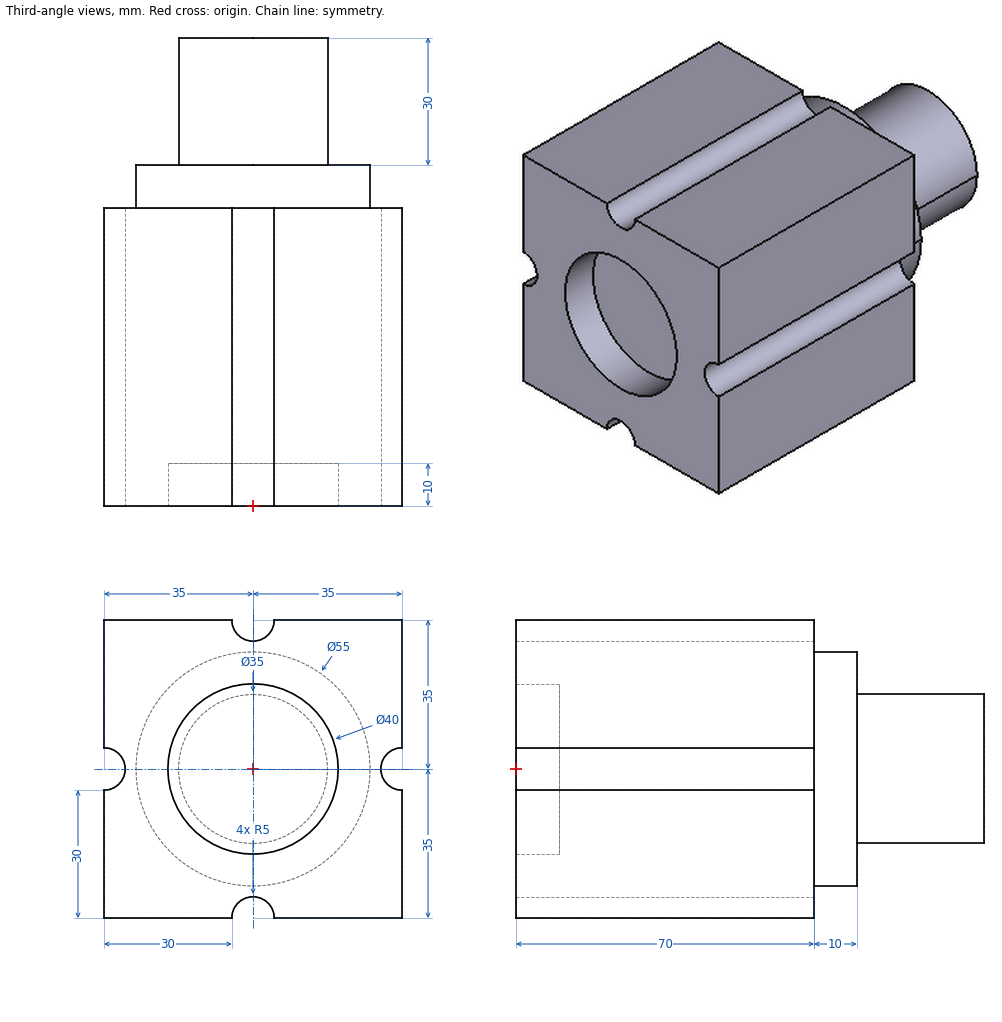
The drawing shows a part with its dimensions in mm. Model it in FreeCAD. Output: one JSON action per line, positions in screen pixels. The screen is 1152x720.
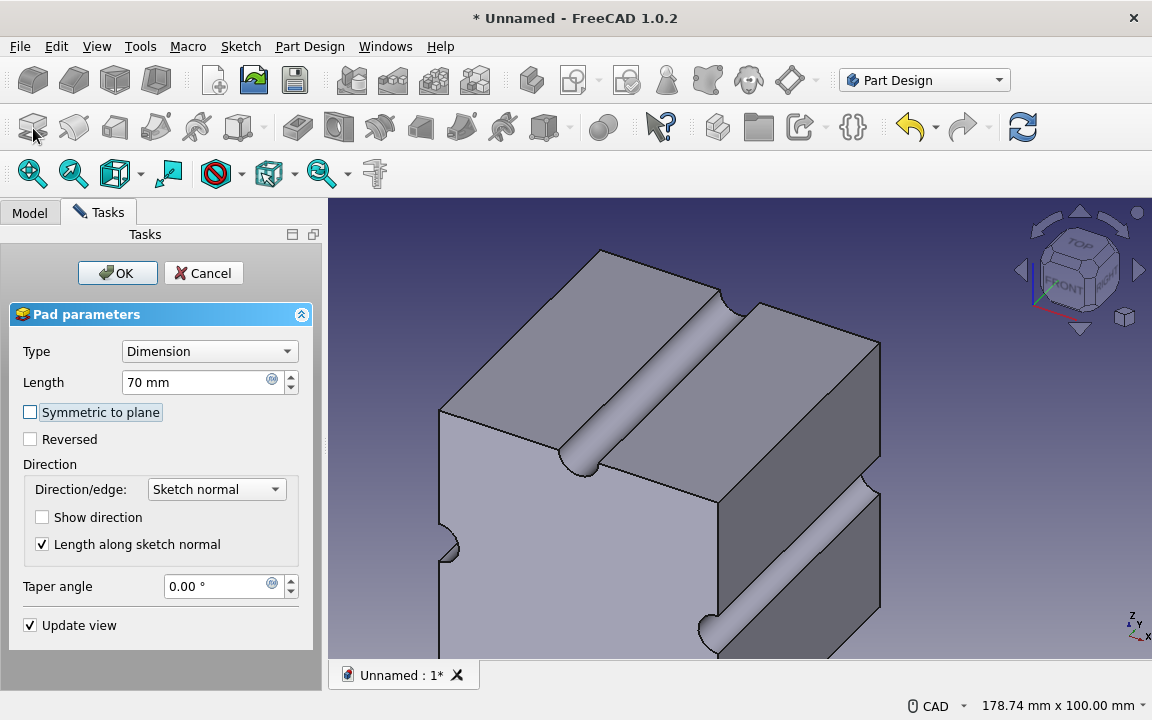
{"action": "left_click", "coordinate": [31, 439]}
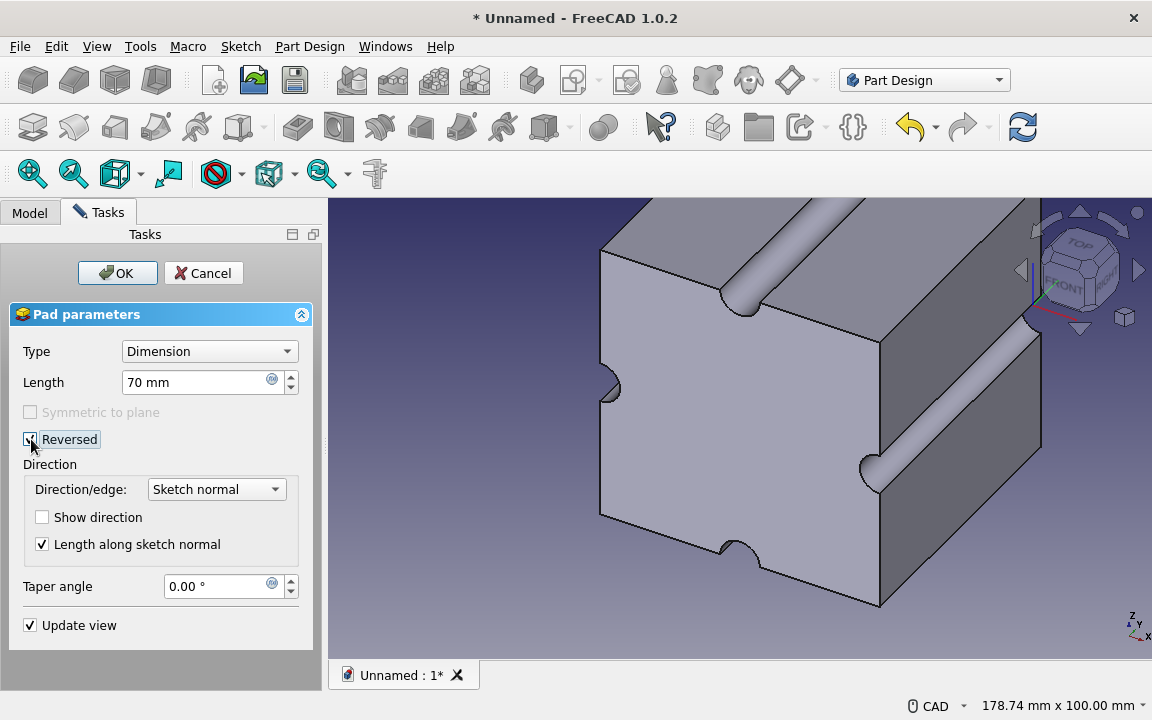
{"action": "left_click", "coordinate": [118, 273]}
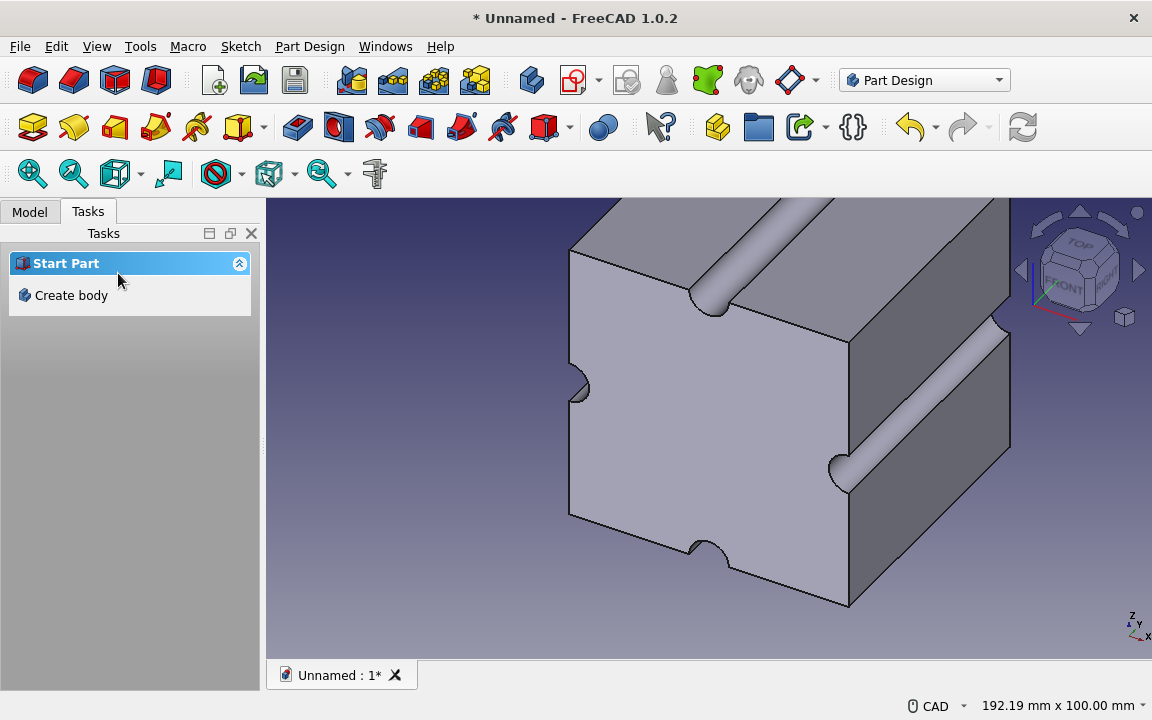
{"action": "key", "text": "v f"}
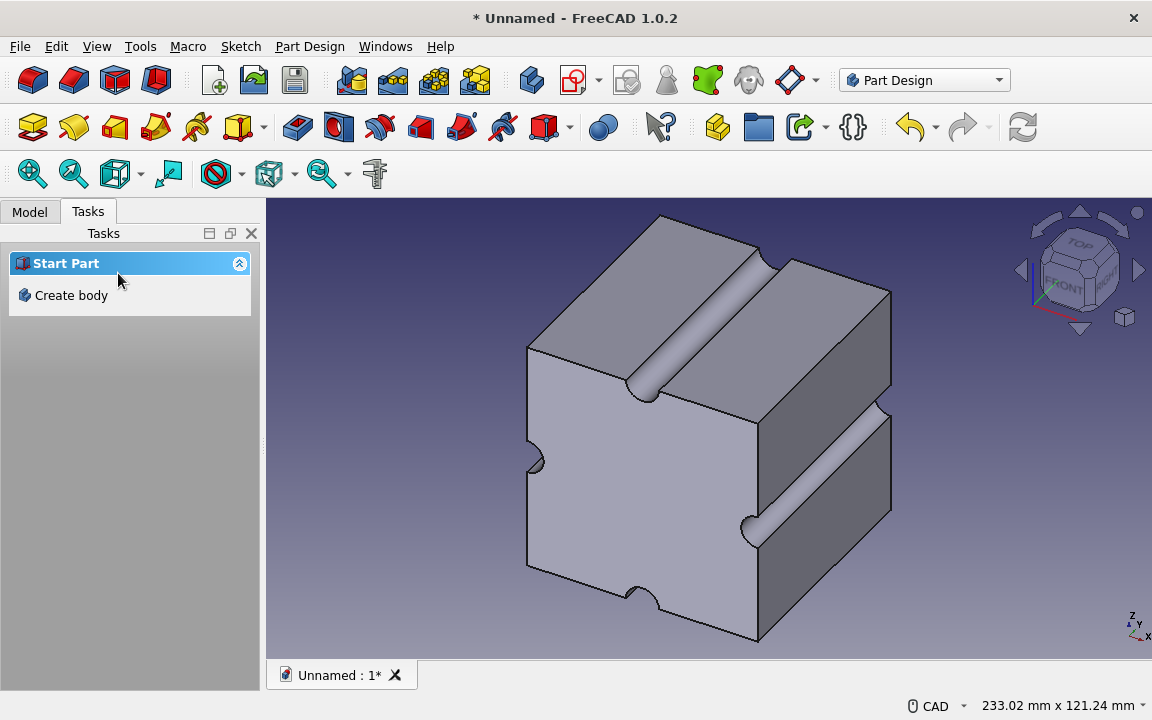
{"action": "left_click", "coordinate": [572, 80]}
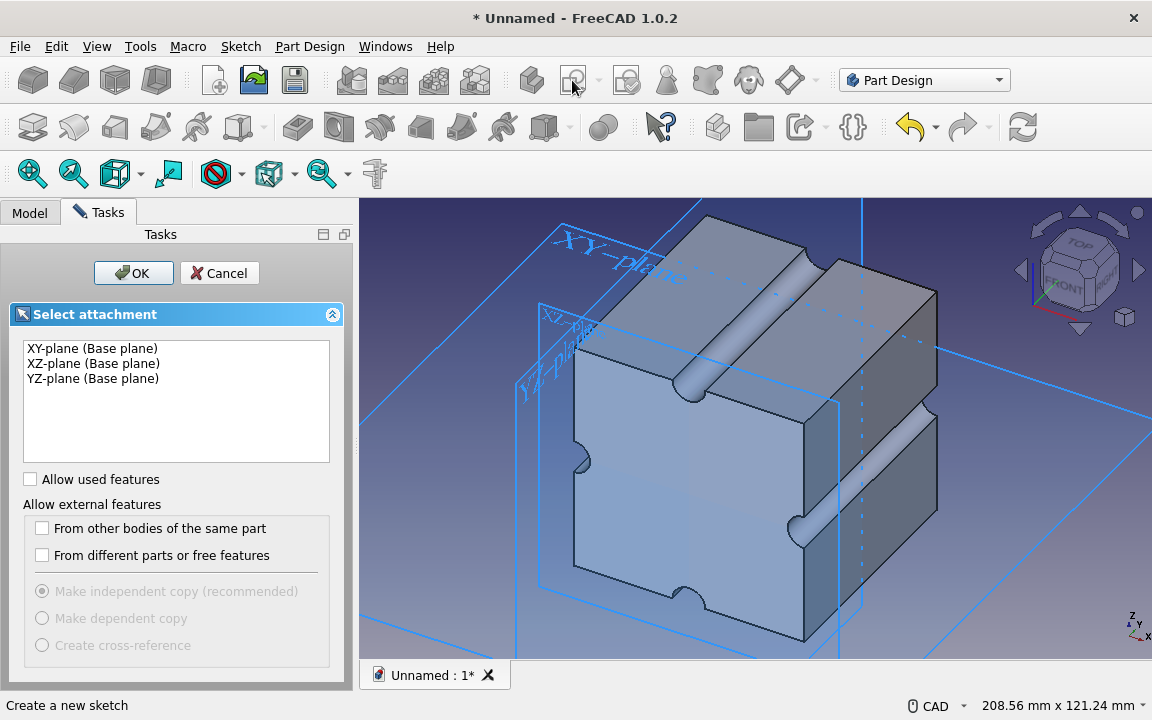
{"action": "left_click", "coordinate": [84, 364]}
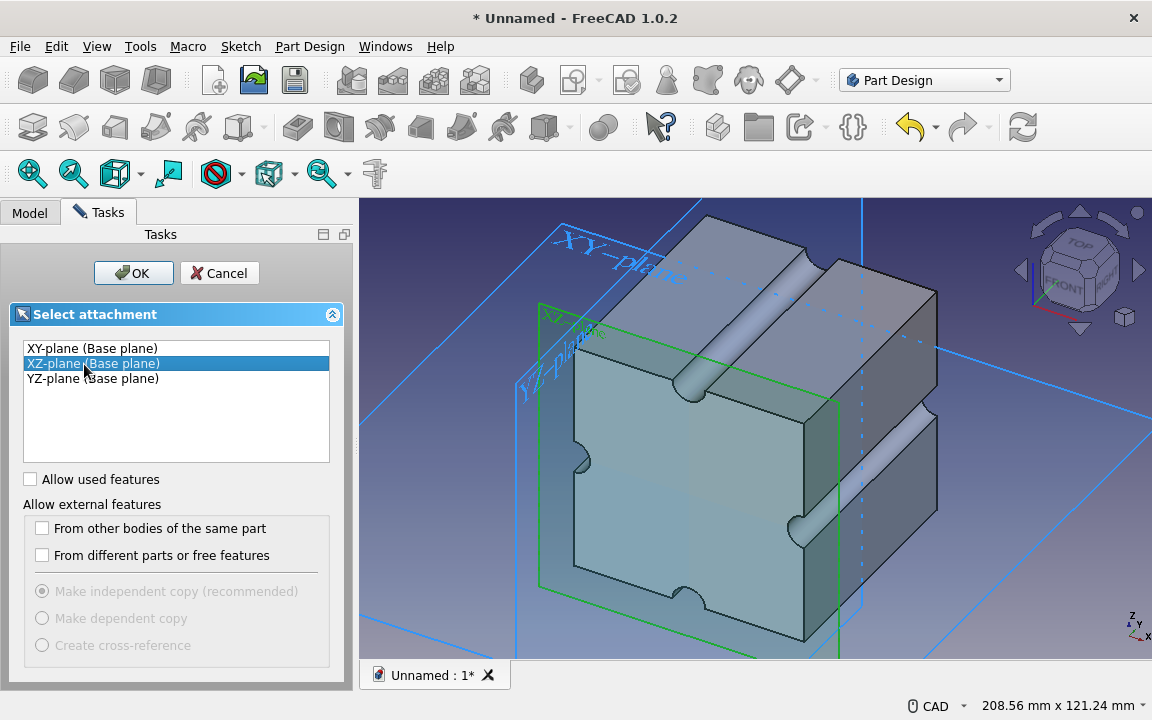
{"action": "left_click", "coordinate": [134, 273]}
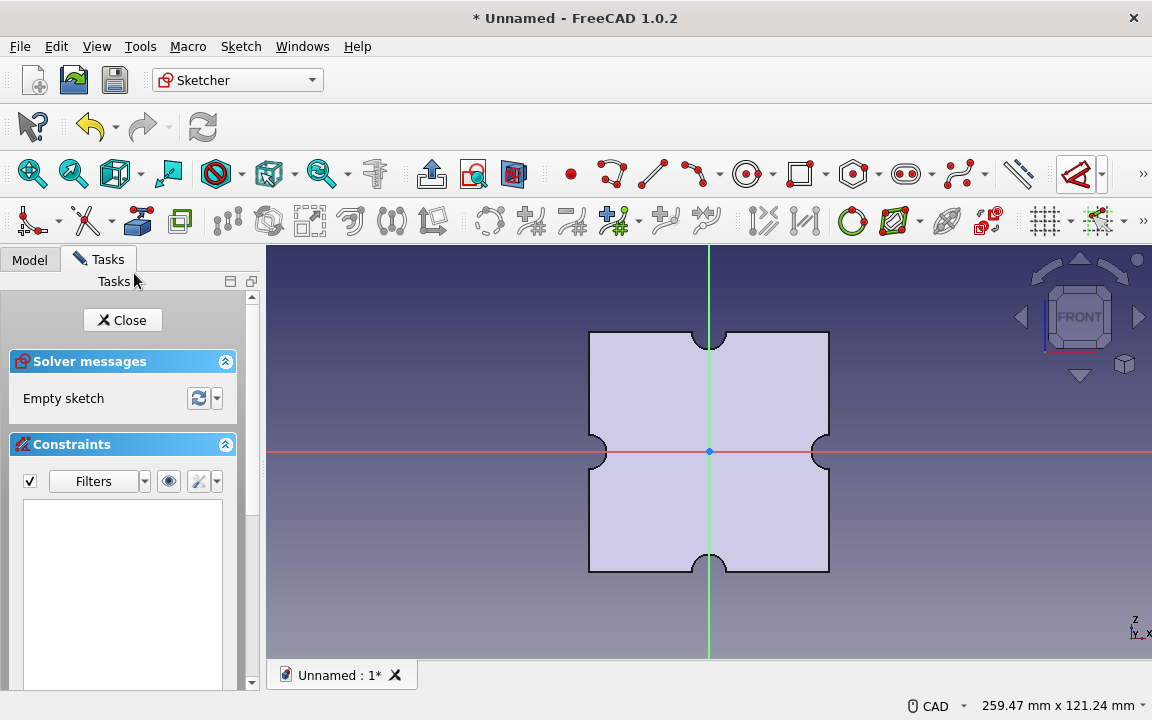
{"action": "scroll", "coordinate": [792, 452], "scroll_direction": "up", "scroll_amount": 3}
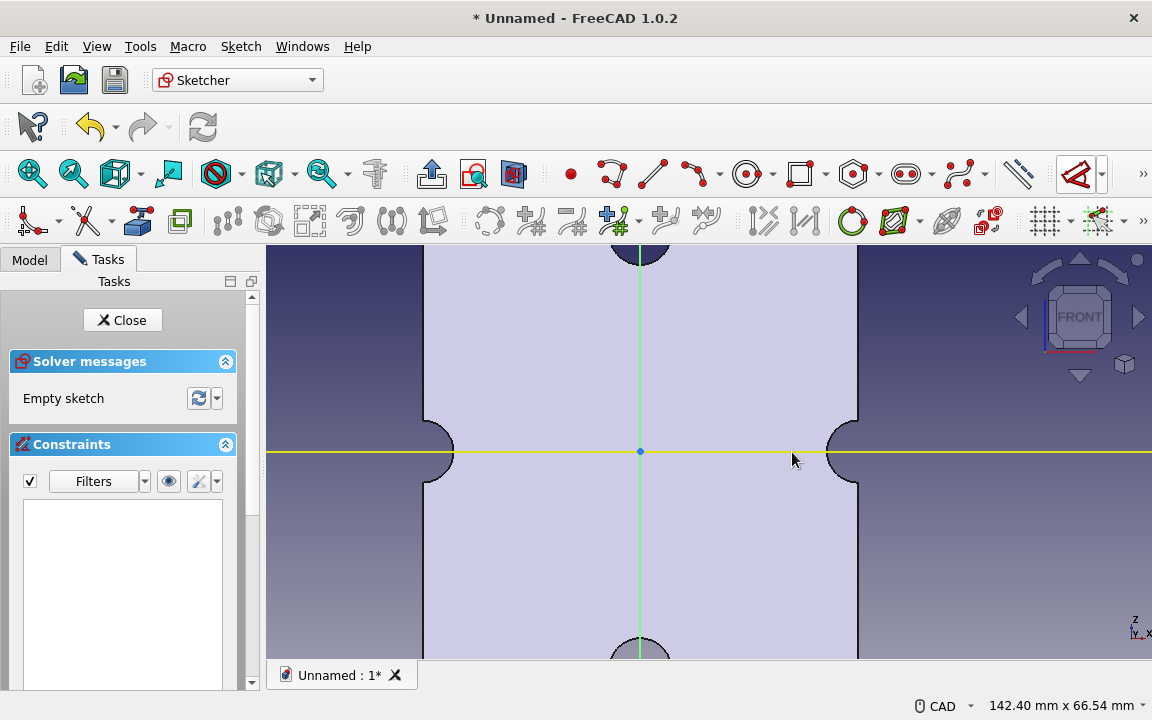
{"action": "left_click", "coordinate": [746, 174]}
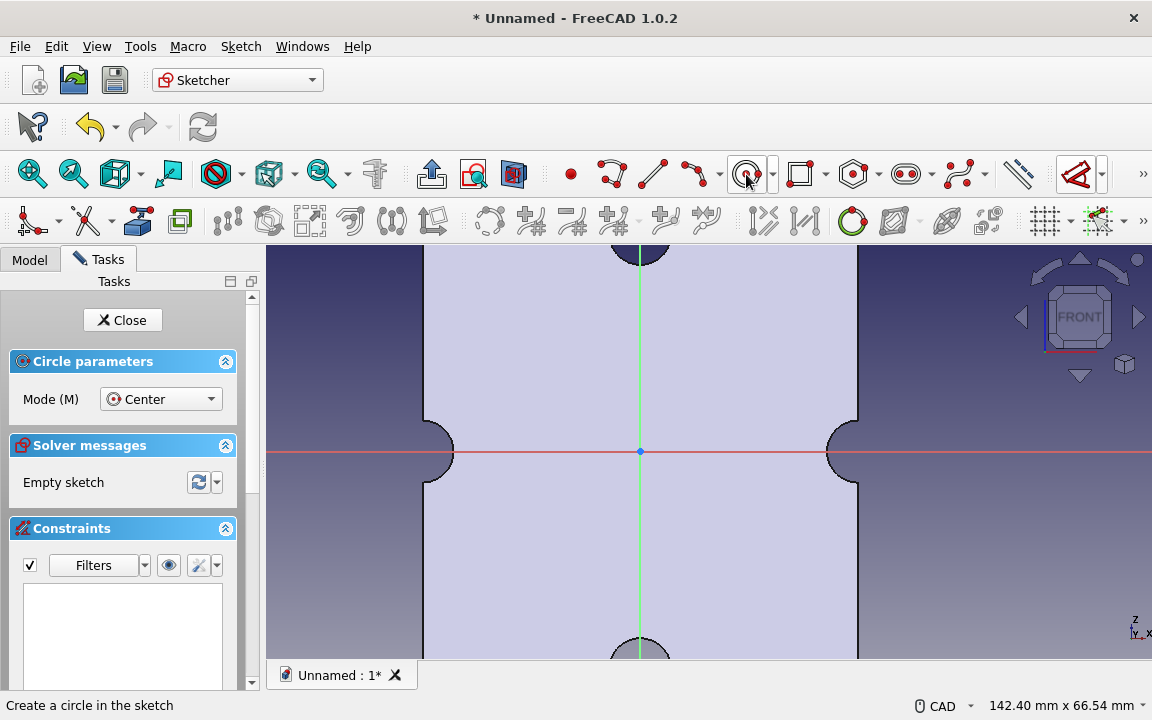
{"action": "left_click", "coordinate": [640, 452]}
{"action": "mouse_move", "coordinate": [728, 364]}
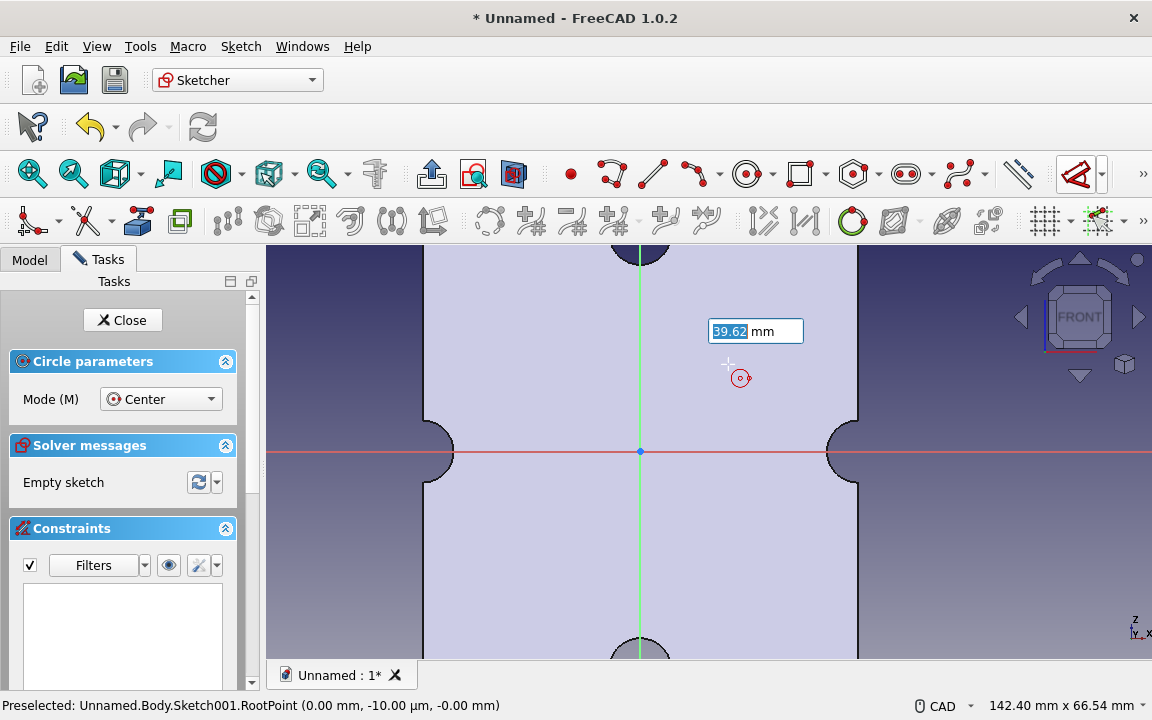
{"action": "type", "text": "40"}
{"action": "key", "text": "Return"}
{"action": "key", "text": "Escape"}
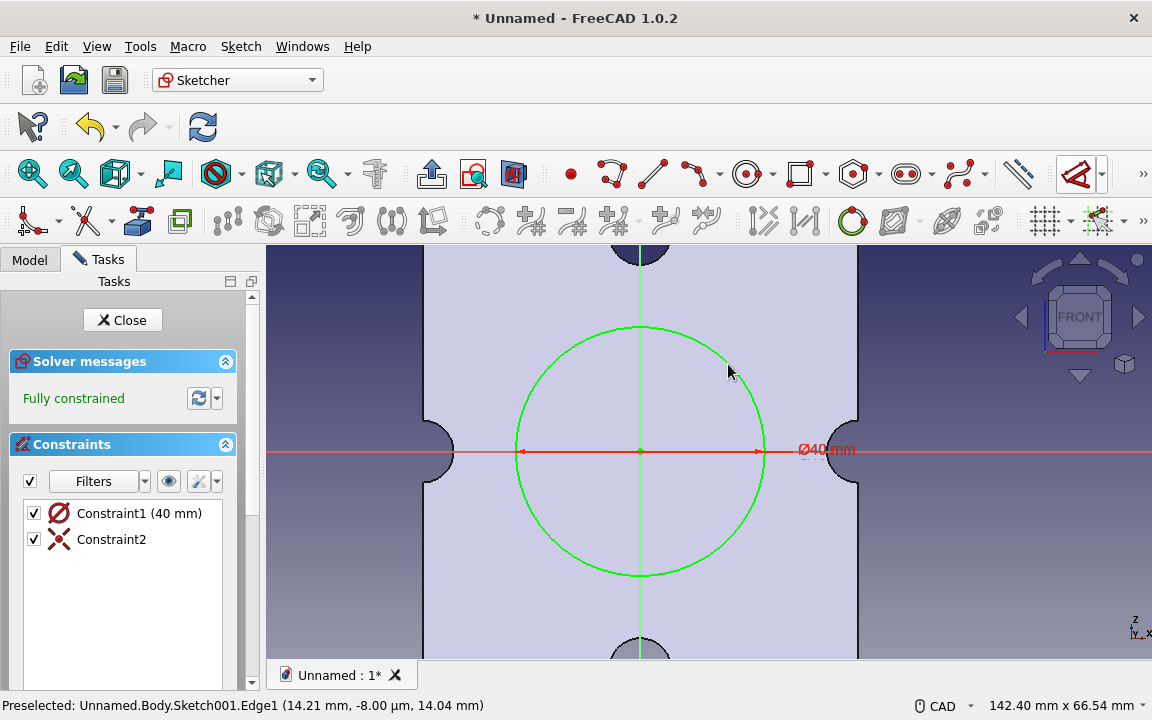
{"action": "left_click", "coordinate": [123, 320]}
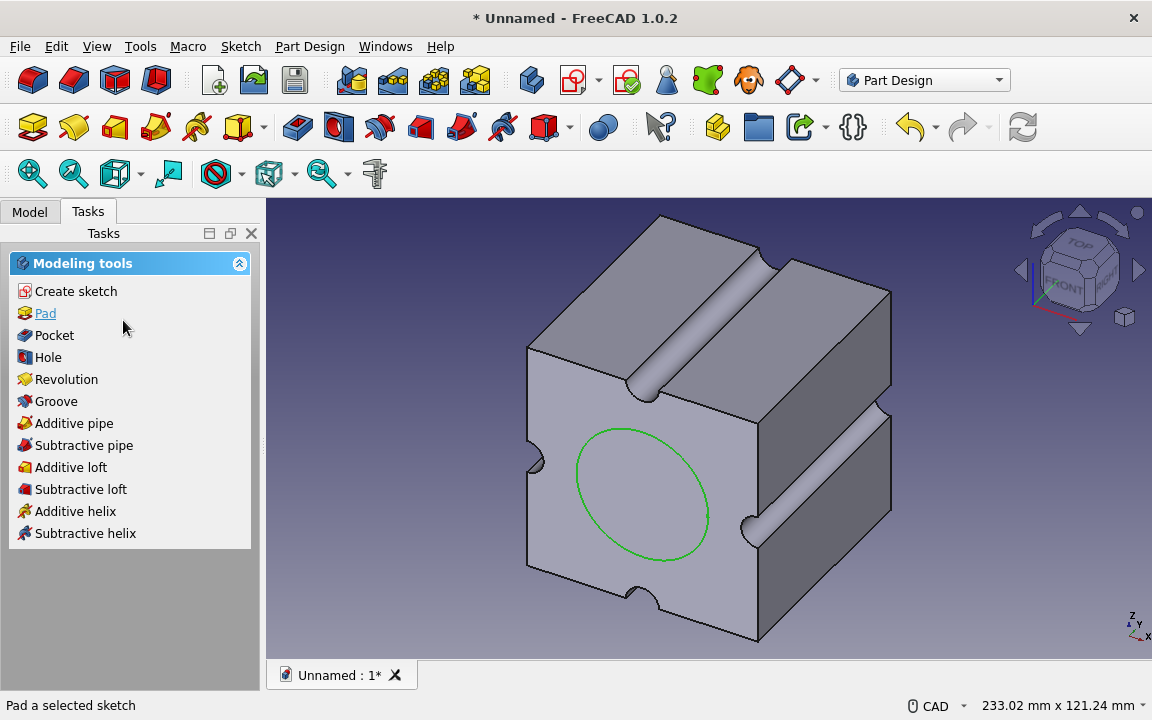
{"action": "left_click", "coordinate": [298, 128]}